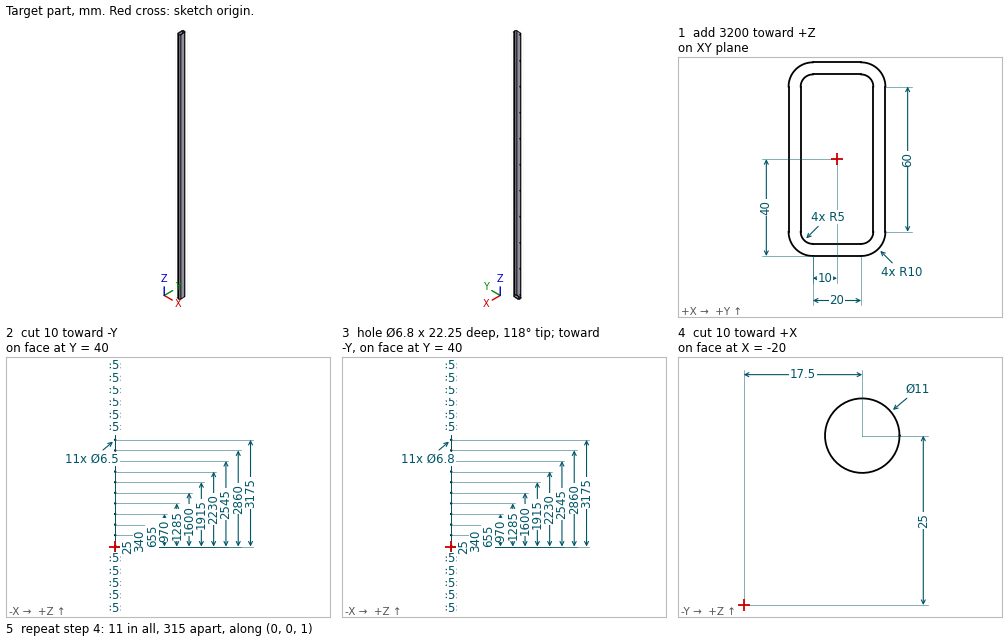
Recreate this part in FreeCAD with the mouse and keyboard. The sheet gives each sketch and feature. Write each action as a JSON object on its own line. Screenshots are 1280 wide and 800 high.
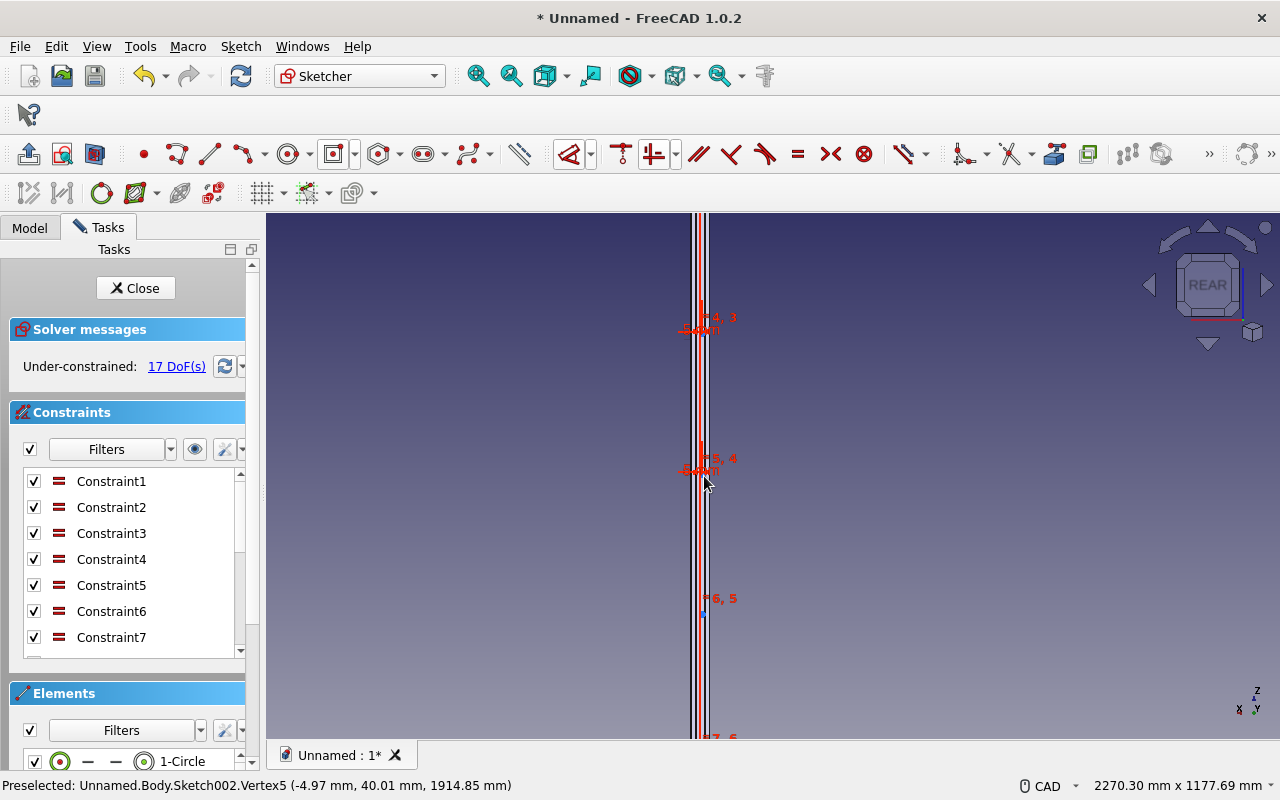
{"action": "scroll", "coordinate": [705, 429], "scroll_direction": "down", "scroll_amount": 7}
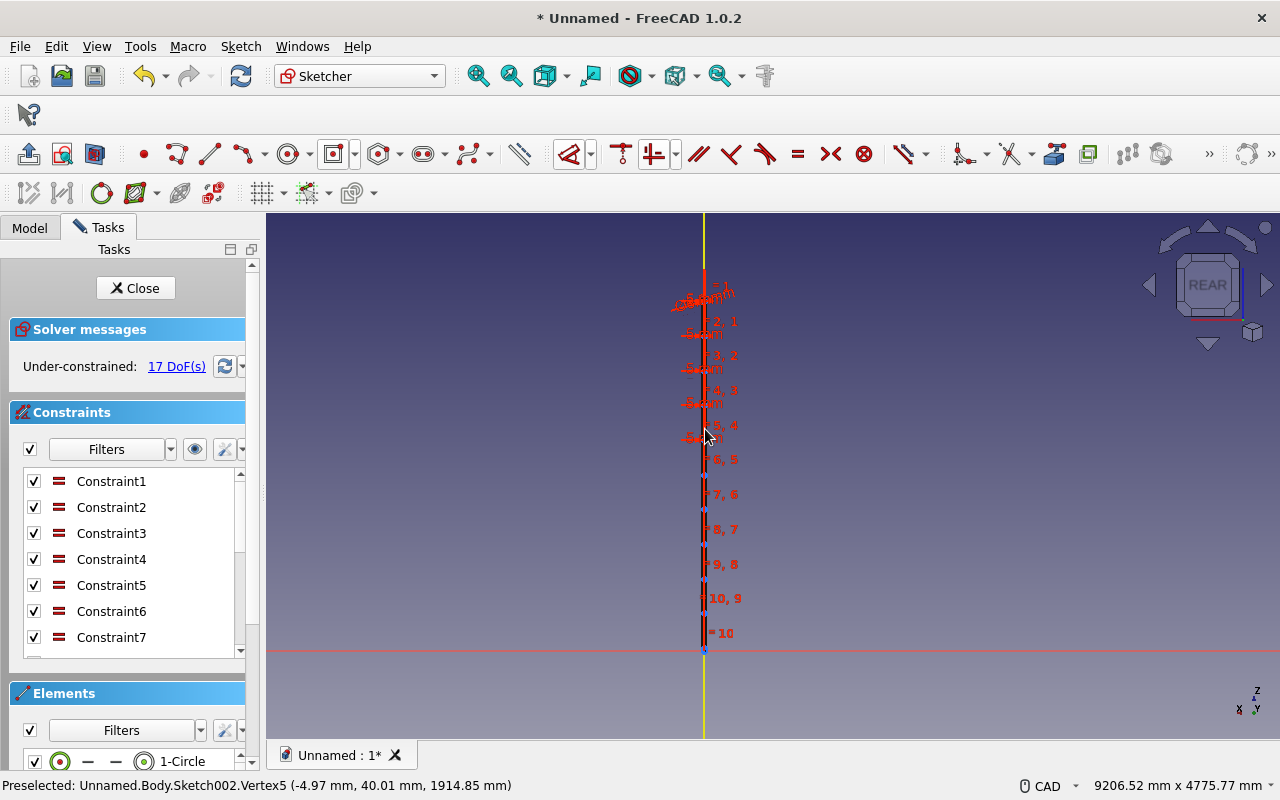
{"action": "scroll", "coordinate": [705, 475], "scroll_direction": "up", "scroll_amount": 22}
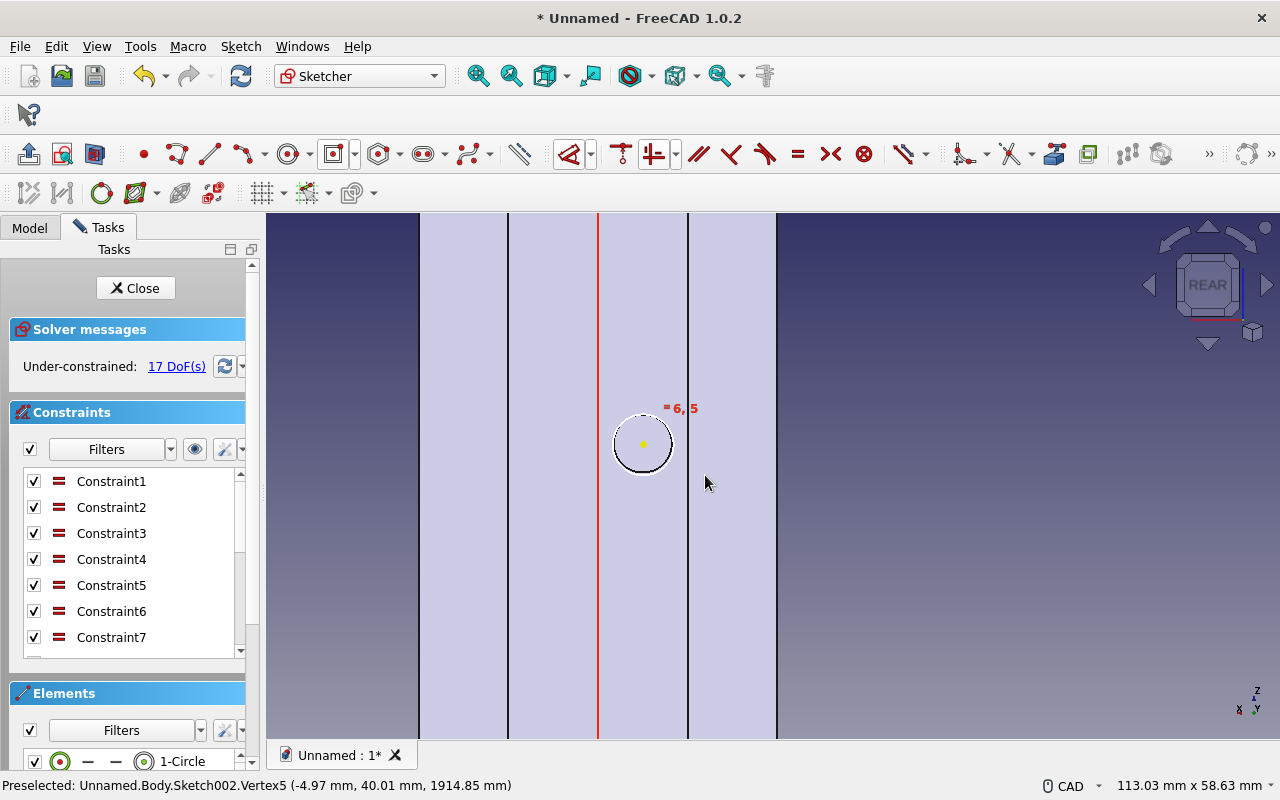
{"action": "left_click", "coordinate": [643, 445]}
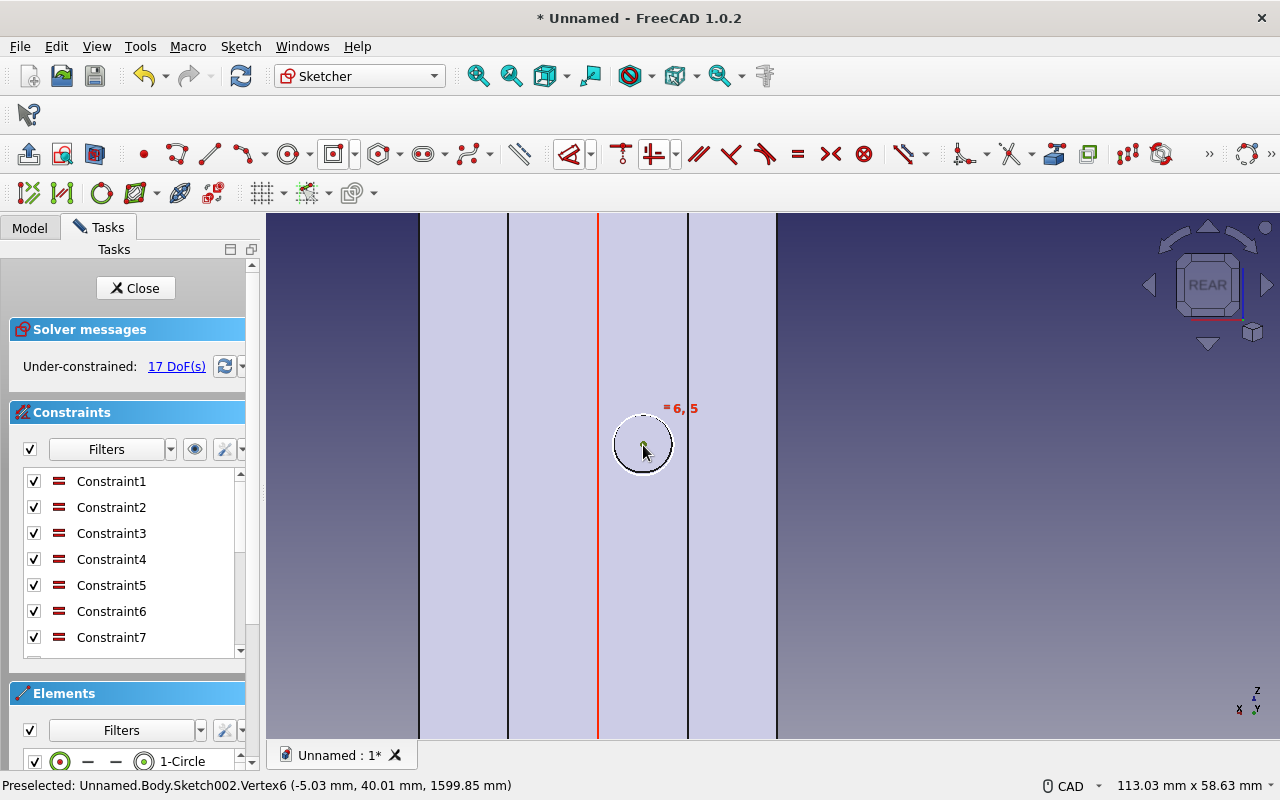
{"action": "key", "text": "l"}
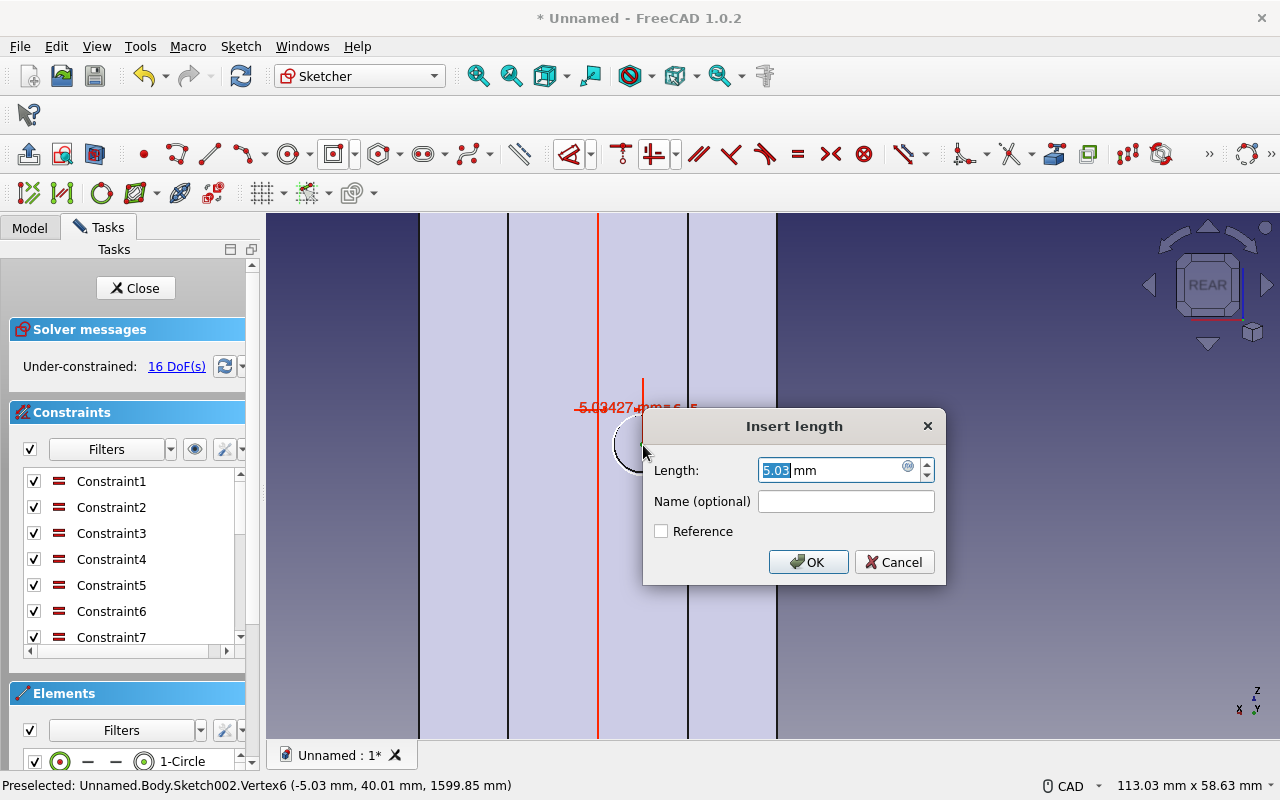
{"action": "type", "text": "5"}
{"action": "key", "text": "Return"}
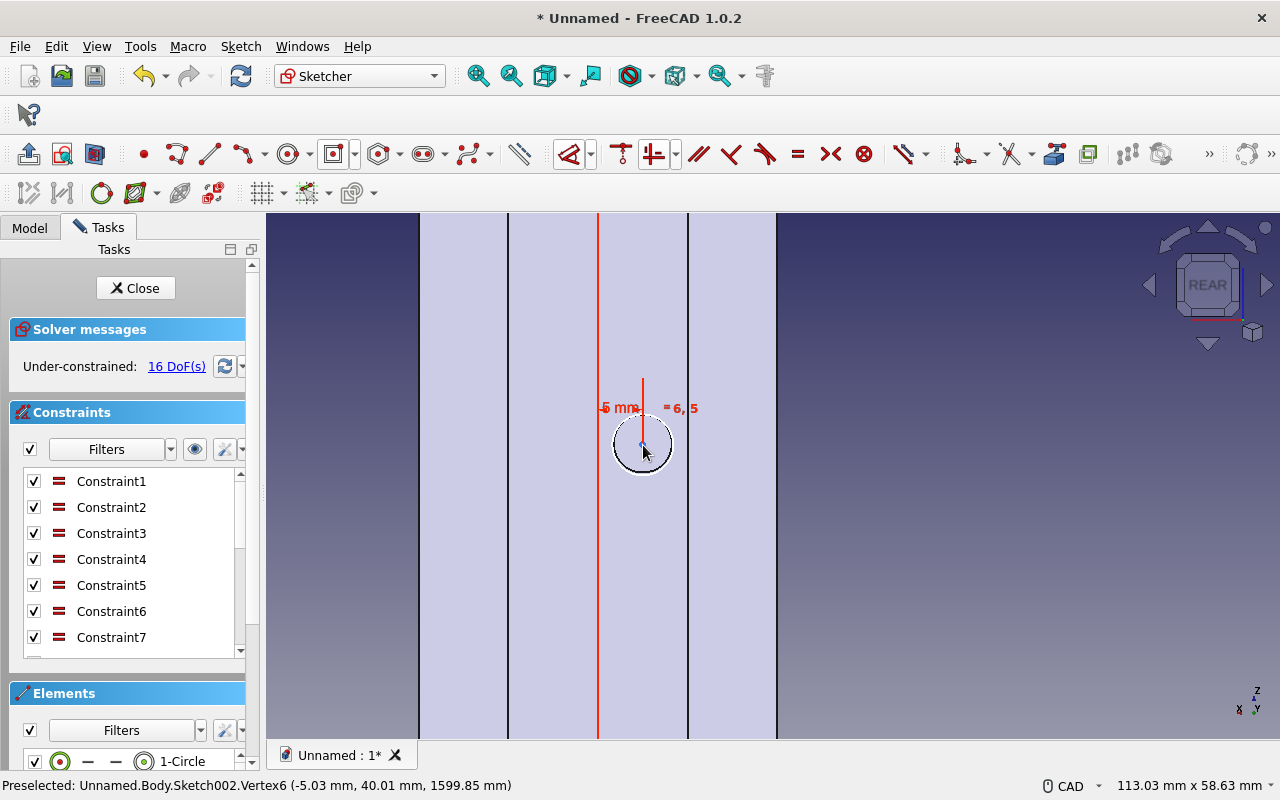
{"action": "scroll", "coordinate": [704, 476], "scroll_direction": "down", "scroll_amount": 15}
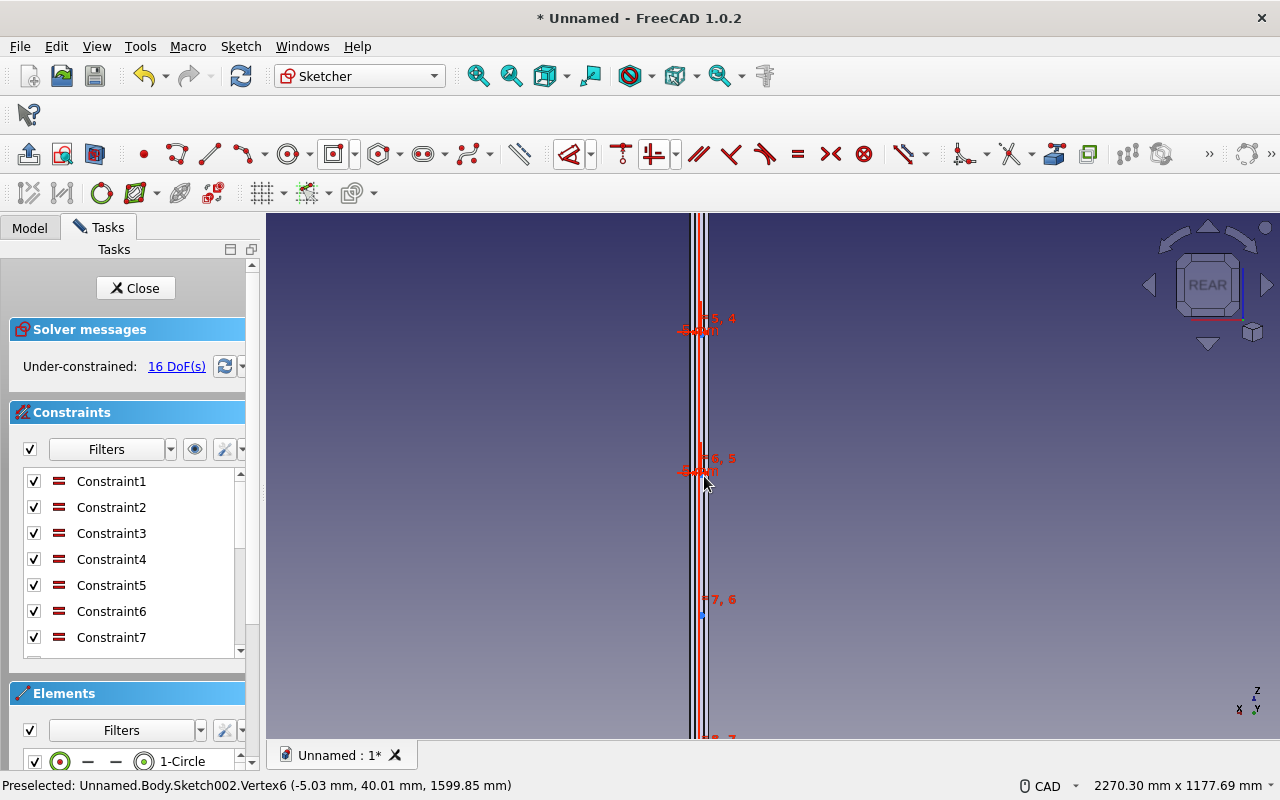
{"action": "scroll", "coordinate": [706, 475], "scroll_direction": "down", "scroll_amount": 7}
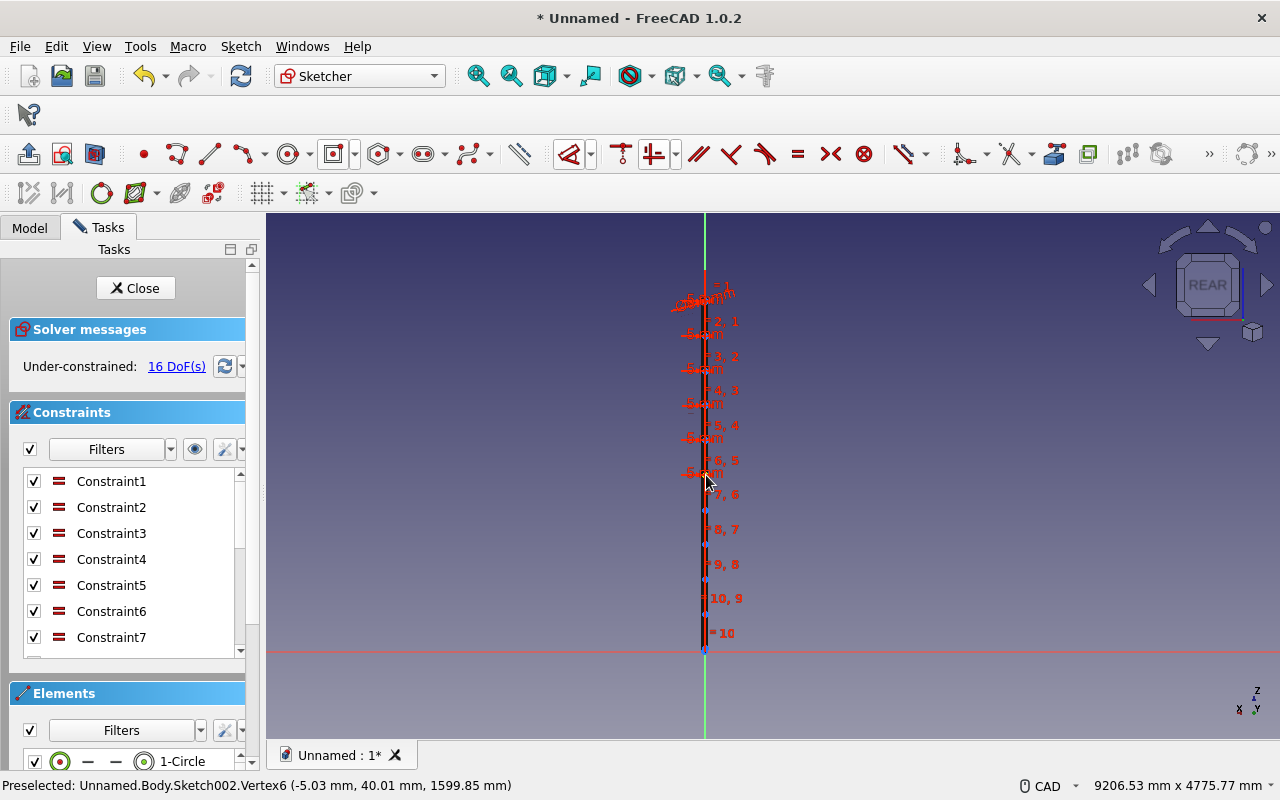
{"action": "scroll", "coordinate": [705, 510], "scroll_direction": "up", "scroll_amount": 22}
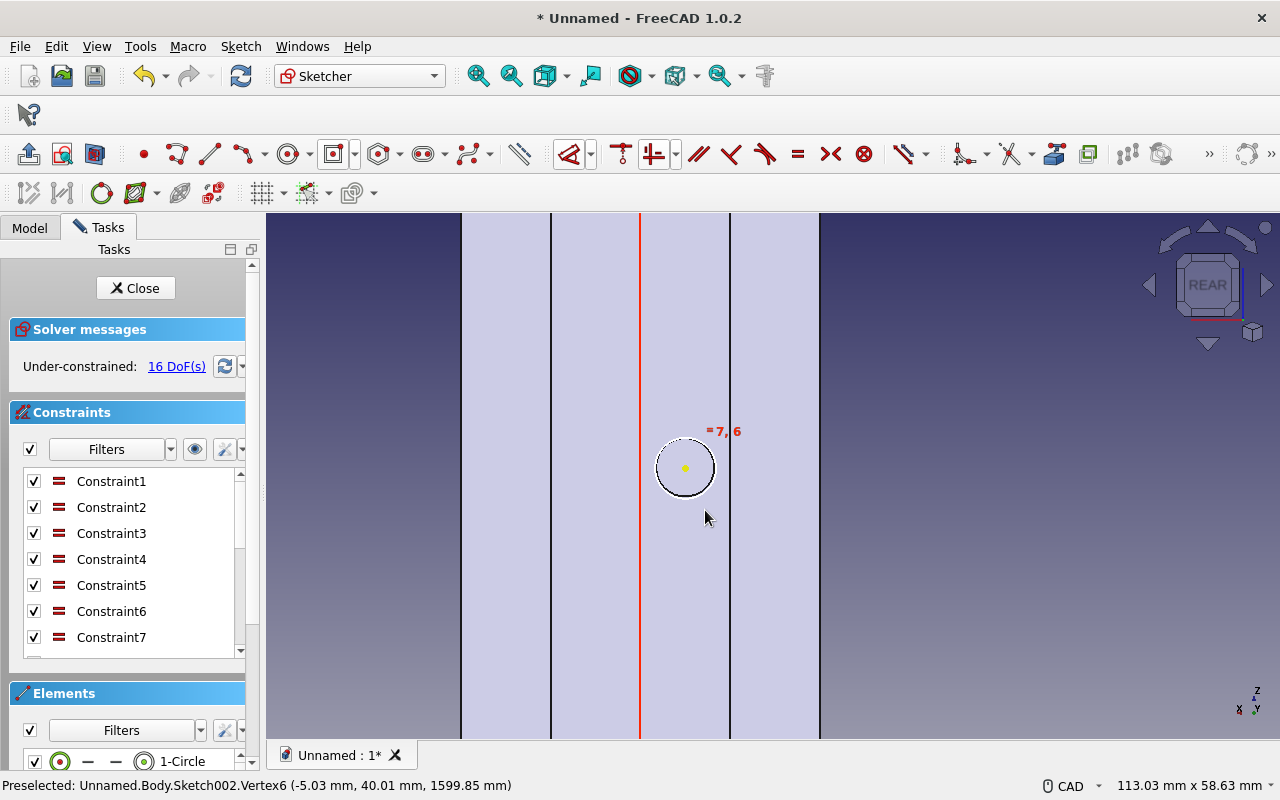
{"action": "left_click", "coordinate": [686, 468]}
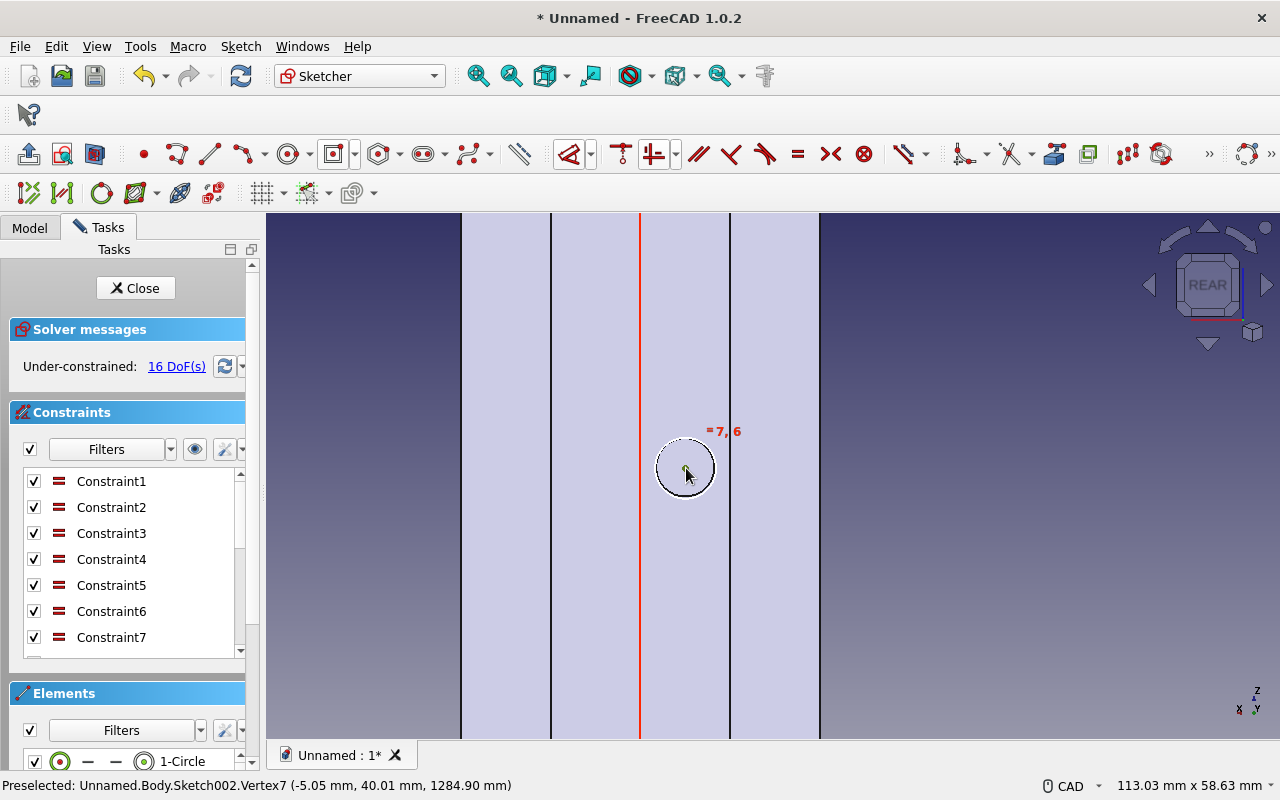
{"action": "left_click", "coordinate": [590, 154]}